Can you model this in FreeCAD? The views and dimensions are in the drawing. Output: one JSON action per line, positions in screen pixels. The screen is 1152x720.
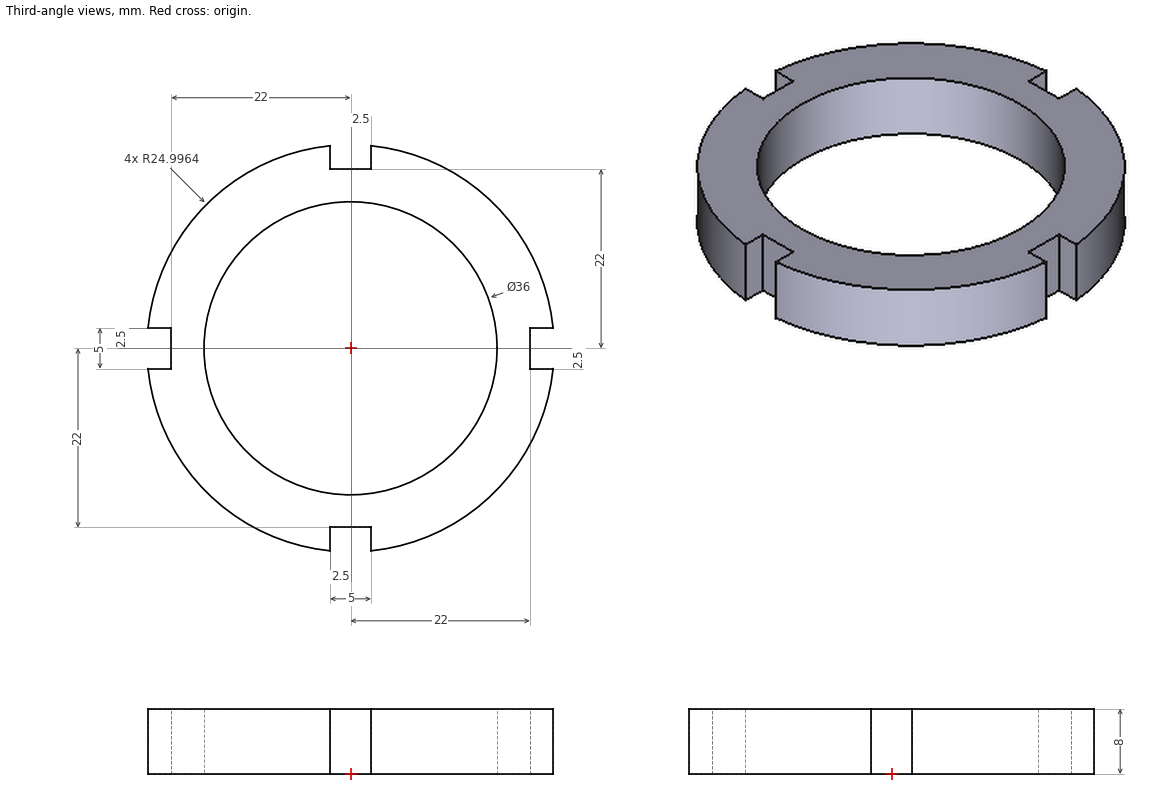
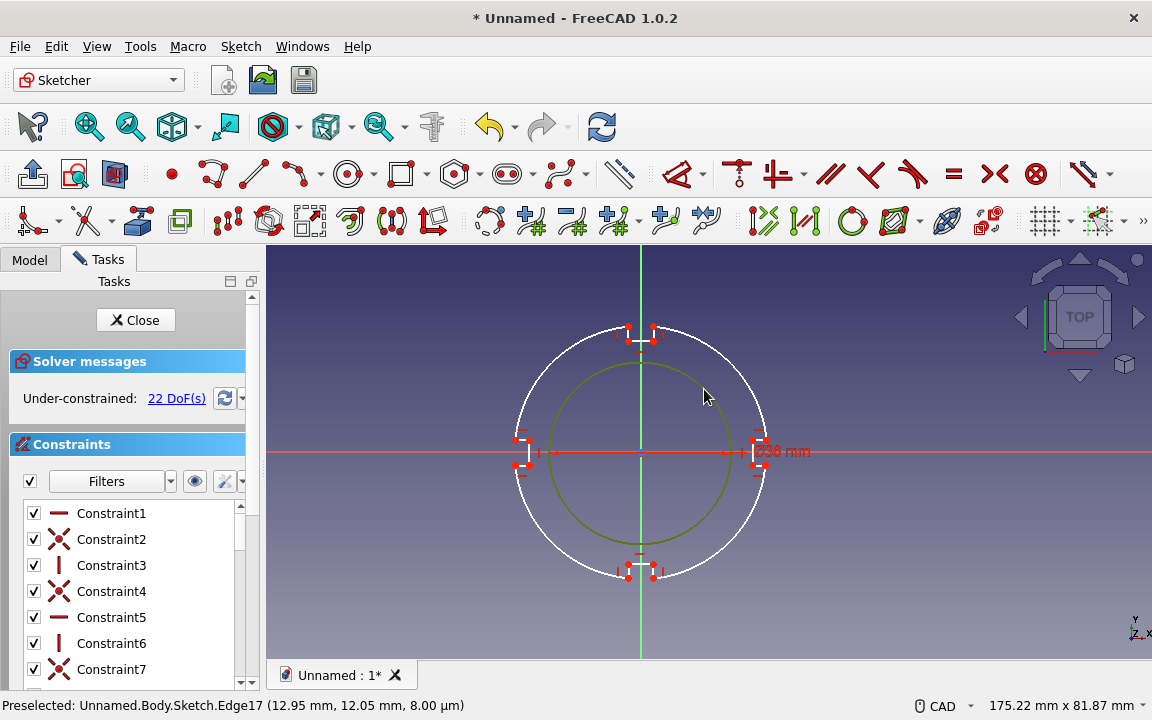
{"action": "left_click", "coordinate": [751, 391]}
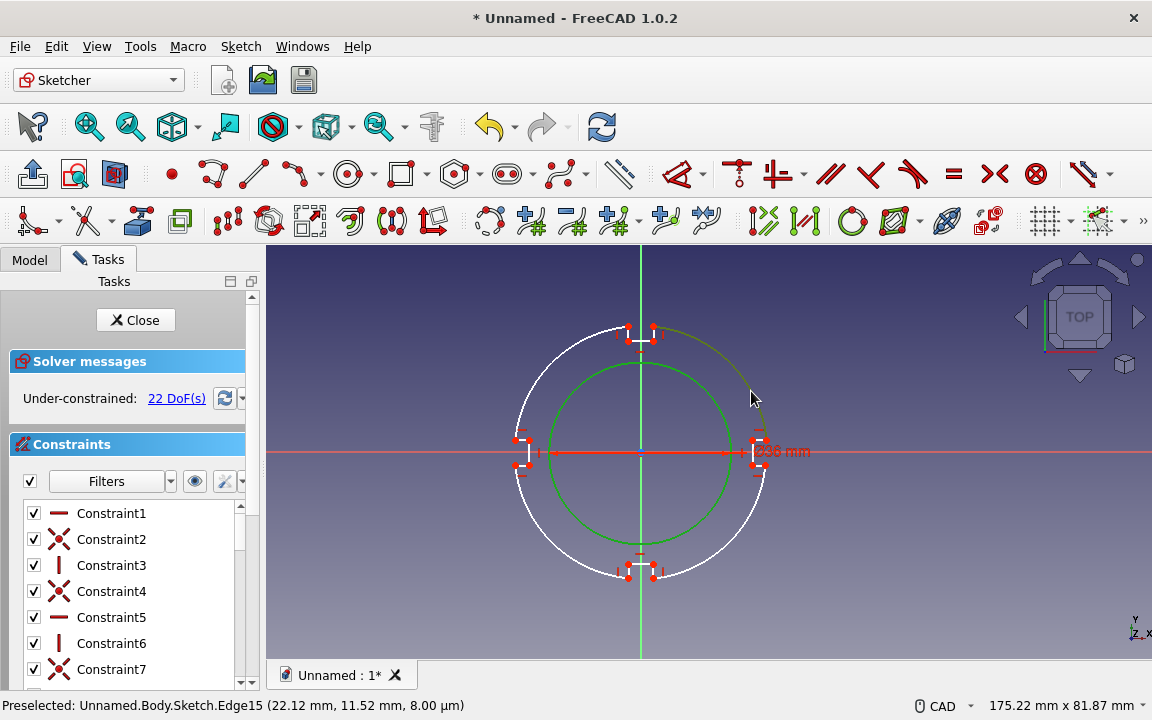
{"action": "key", "text": "c"}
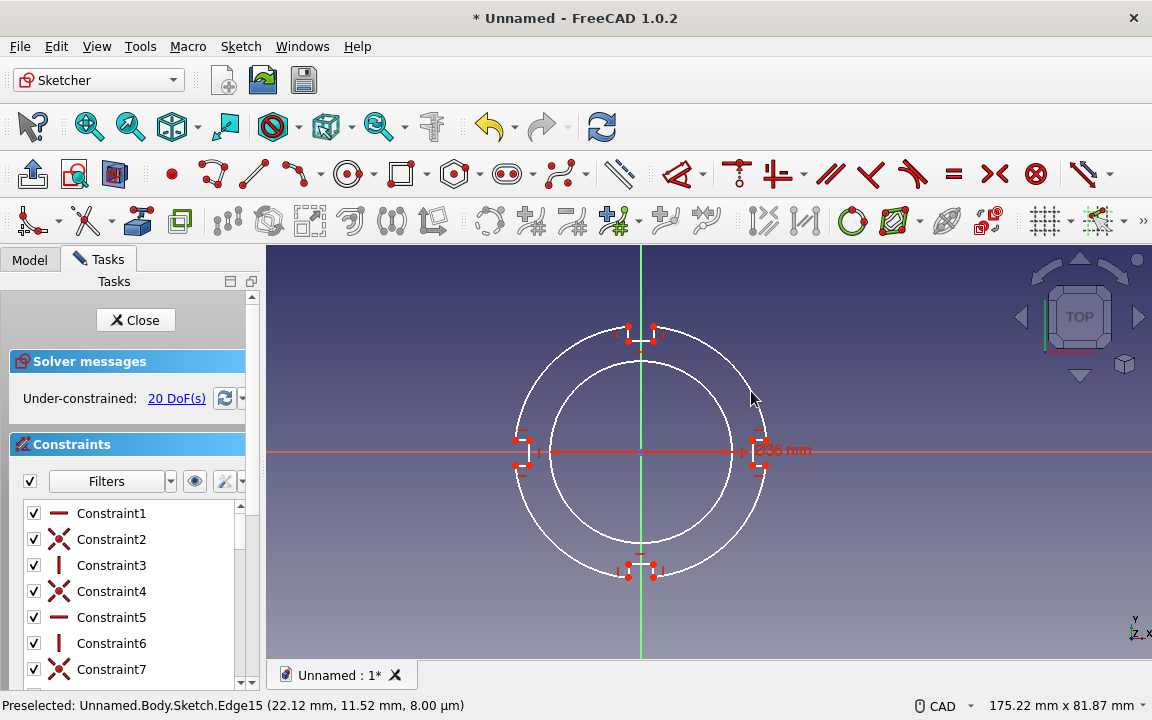
{"action": "left_click", "coordinate": [705, 388]}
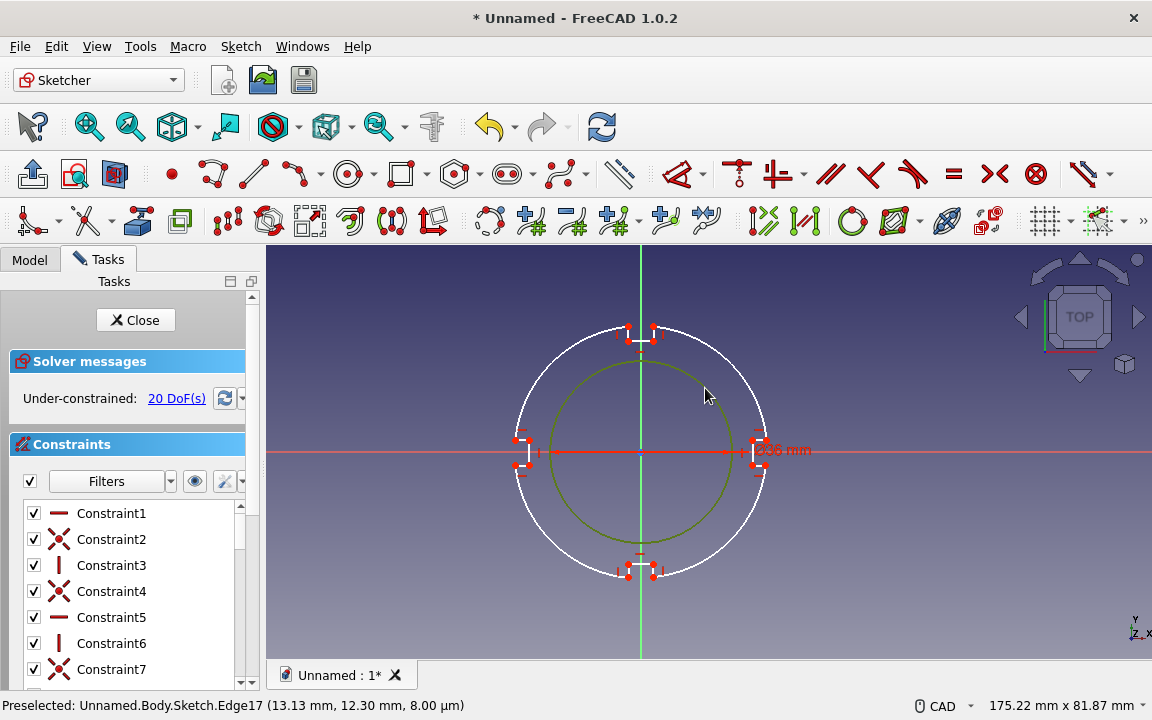
{"action": "left_click", "coordinate": [579, 342]}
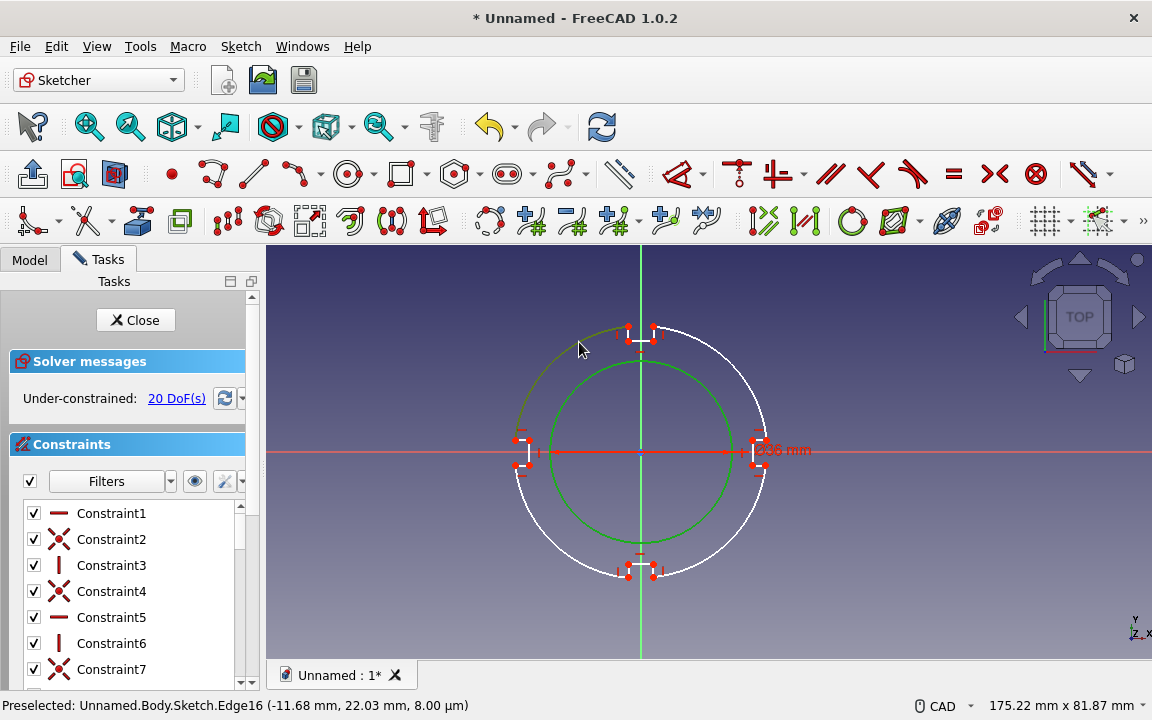
{"action": "key", "text": "c"}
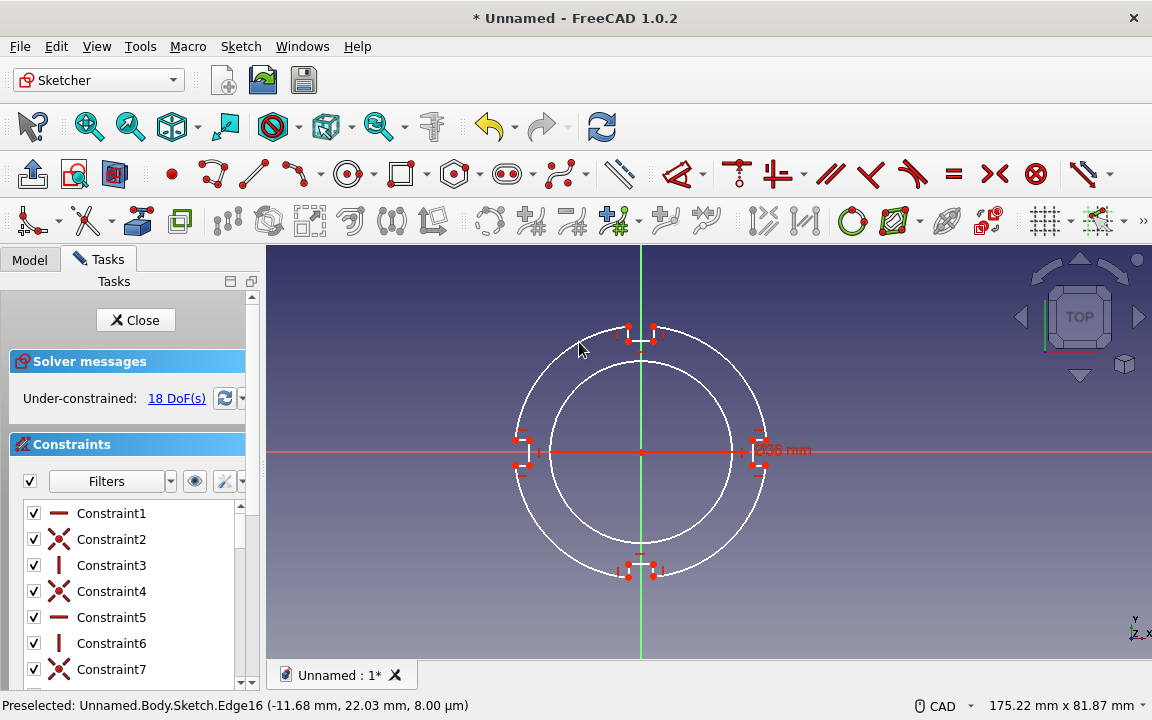
{"action": "left_click_drag", "start_coordinate": [631, 442], "coordinate": [651, 462]}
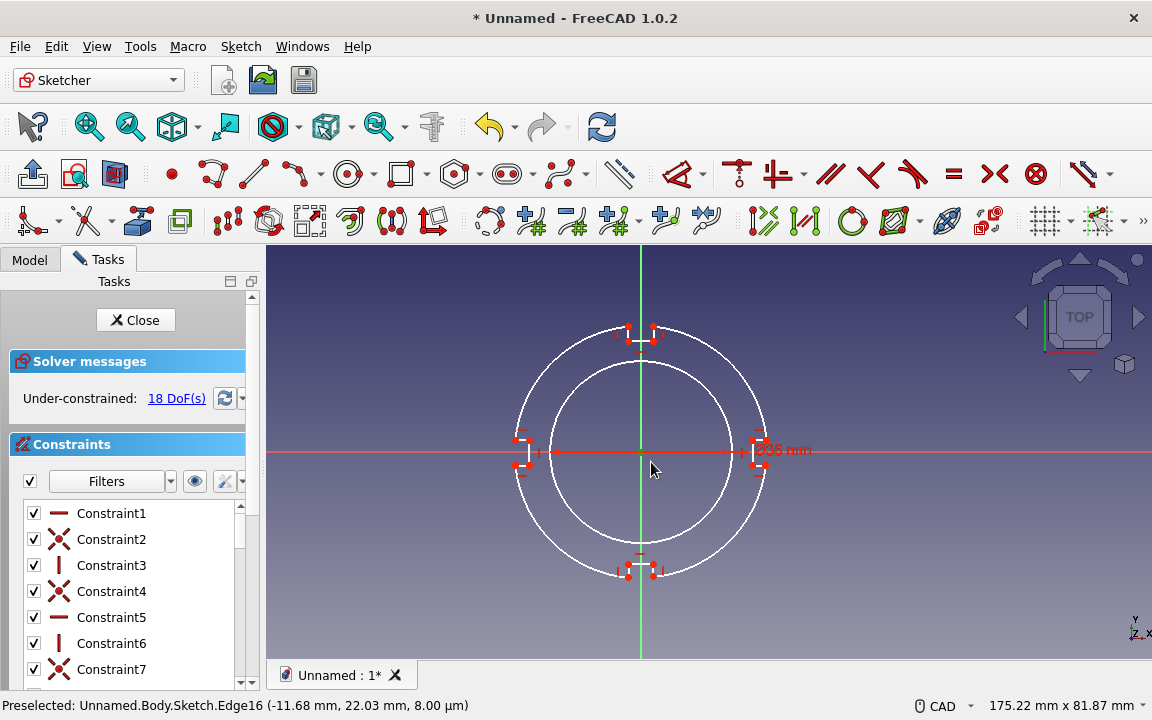
{"action": "left_click", "coordinate": [737, 174]}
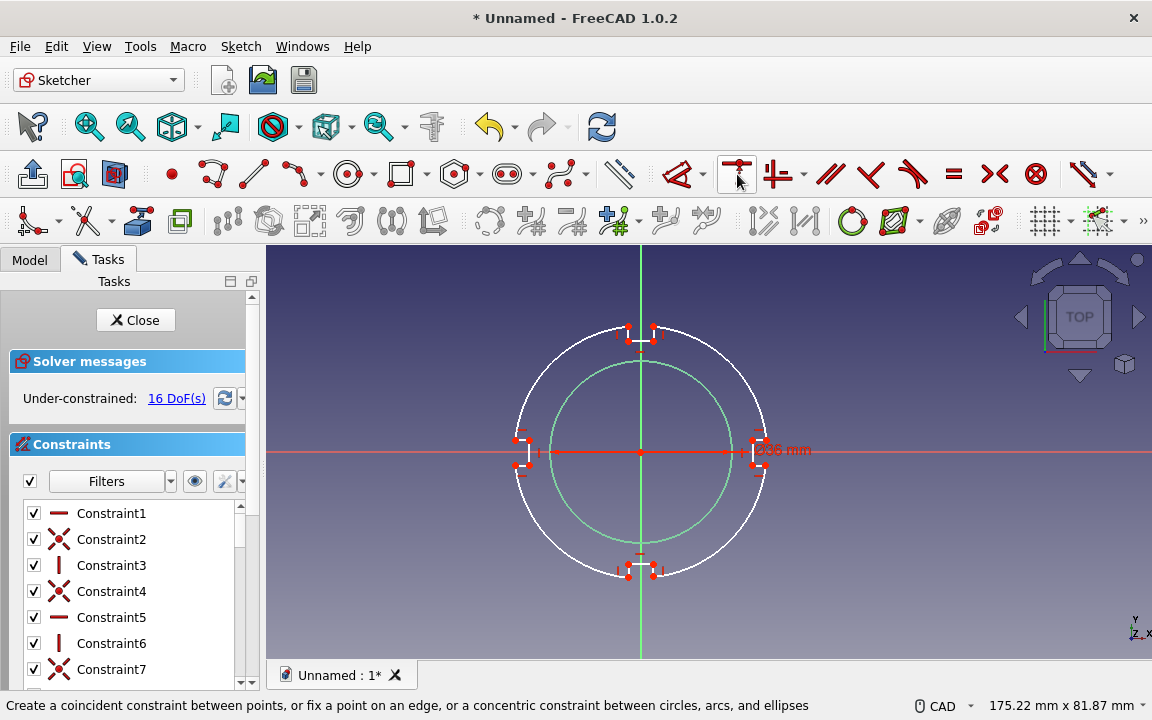
{"action": "left_click", "coordinate": [531, 514]}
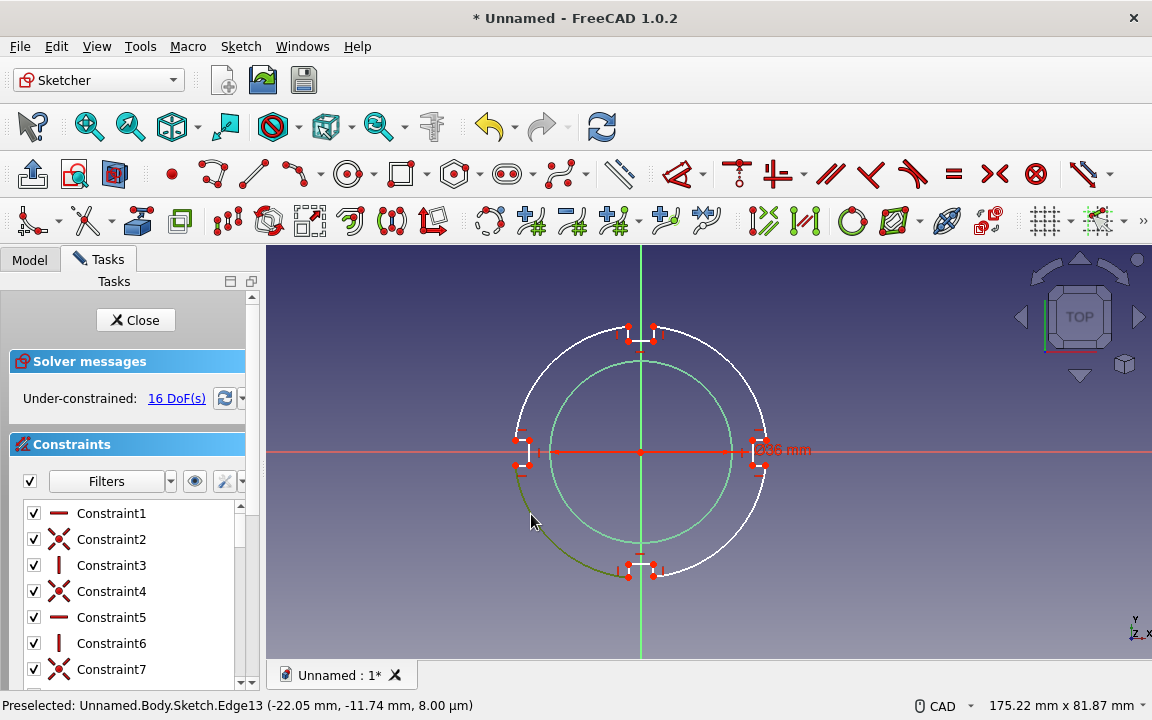
{"action": "left_click", "coordinate": [702, 562]}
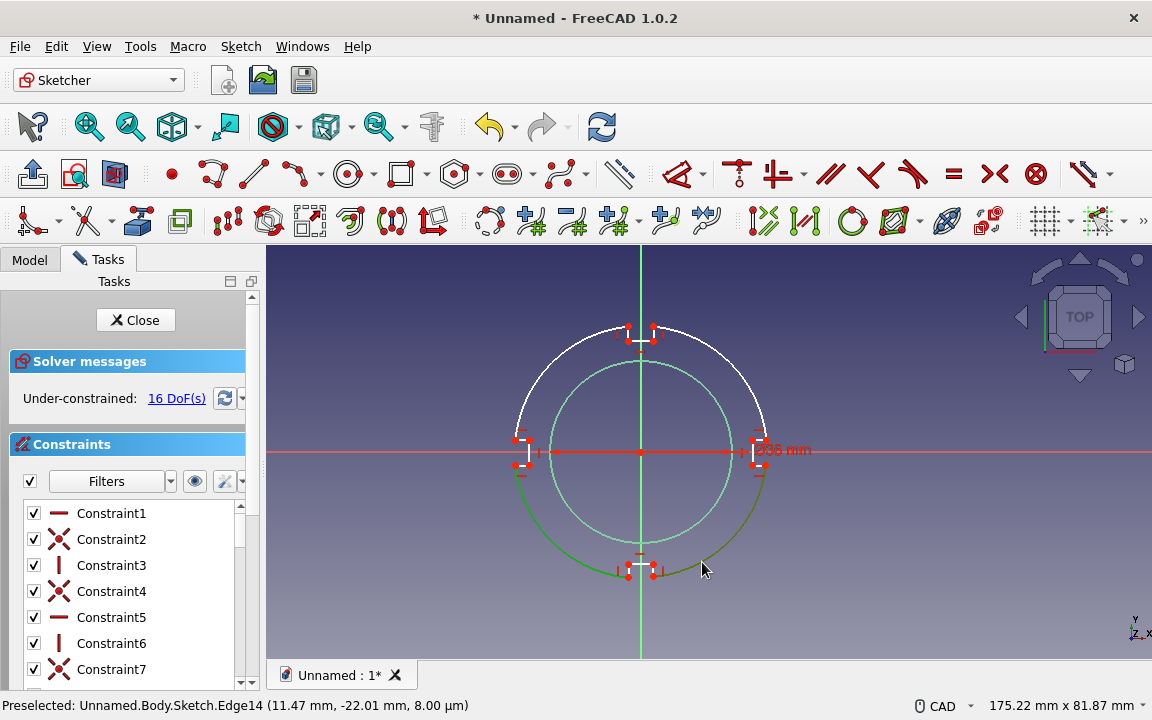
{"action": "left_click", "coordinate": [751, 391]}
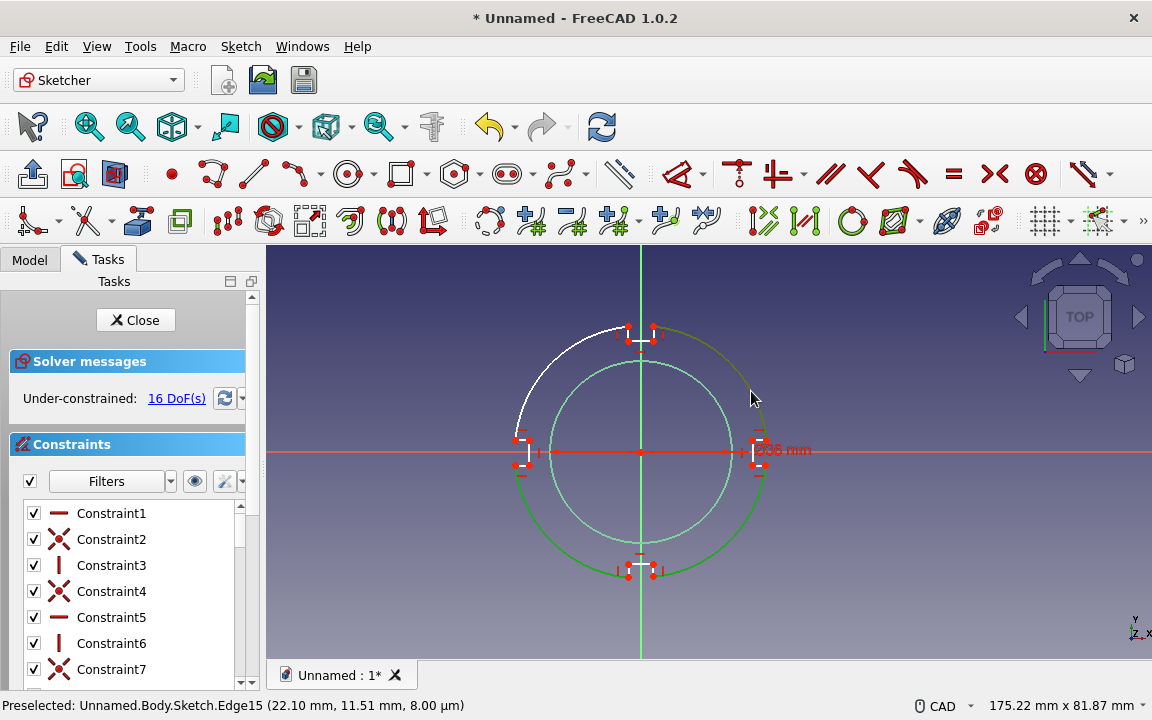
{"action": "left_click", "coordinate": [579, 342]}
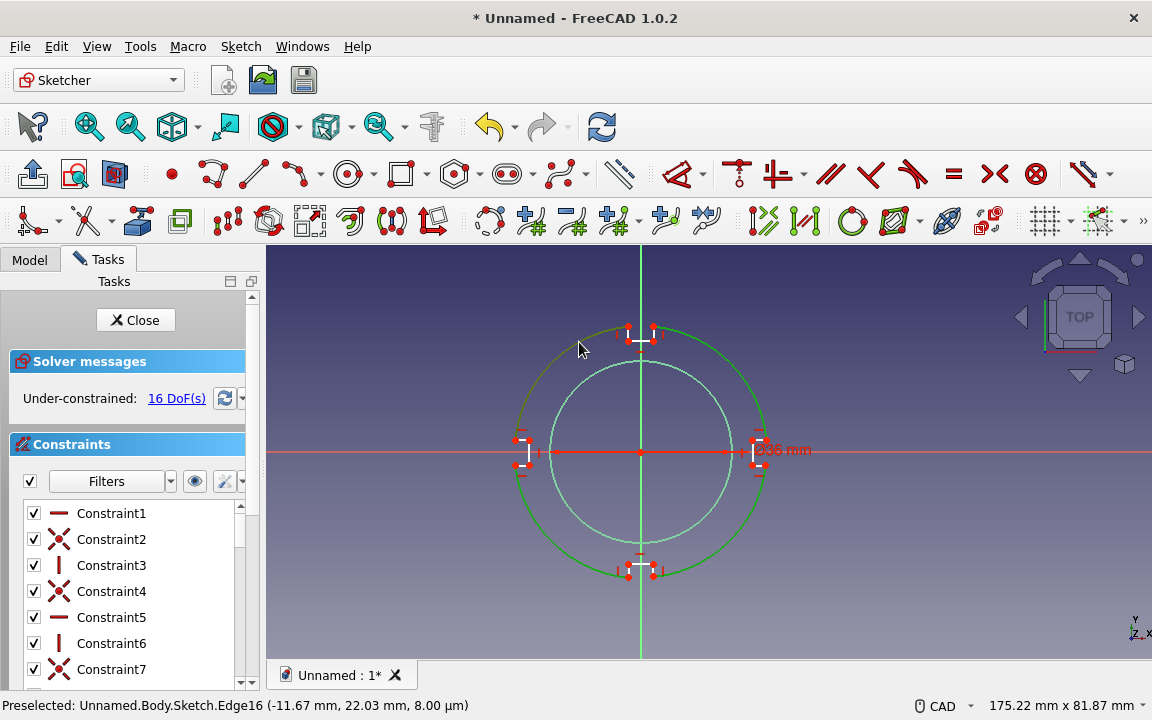
{"action": "key", "text": "e"}